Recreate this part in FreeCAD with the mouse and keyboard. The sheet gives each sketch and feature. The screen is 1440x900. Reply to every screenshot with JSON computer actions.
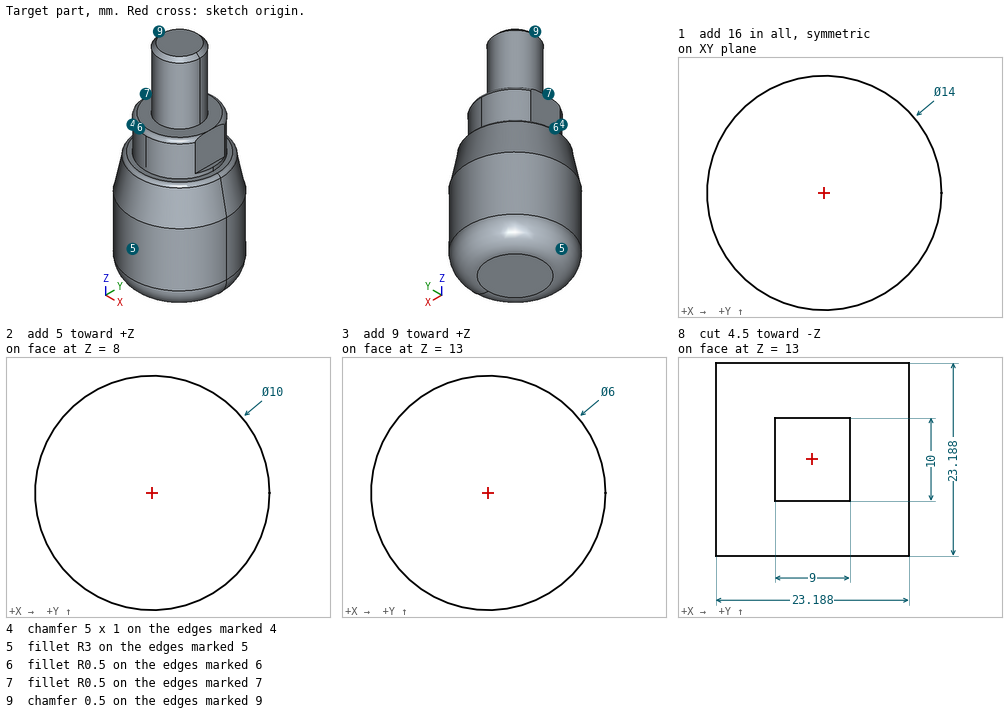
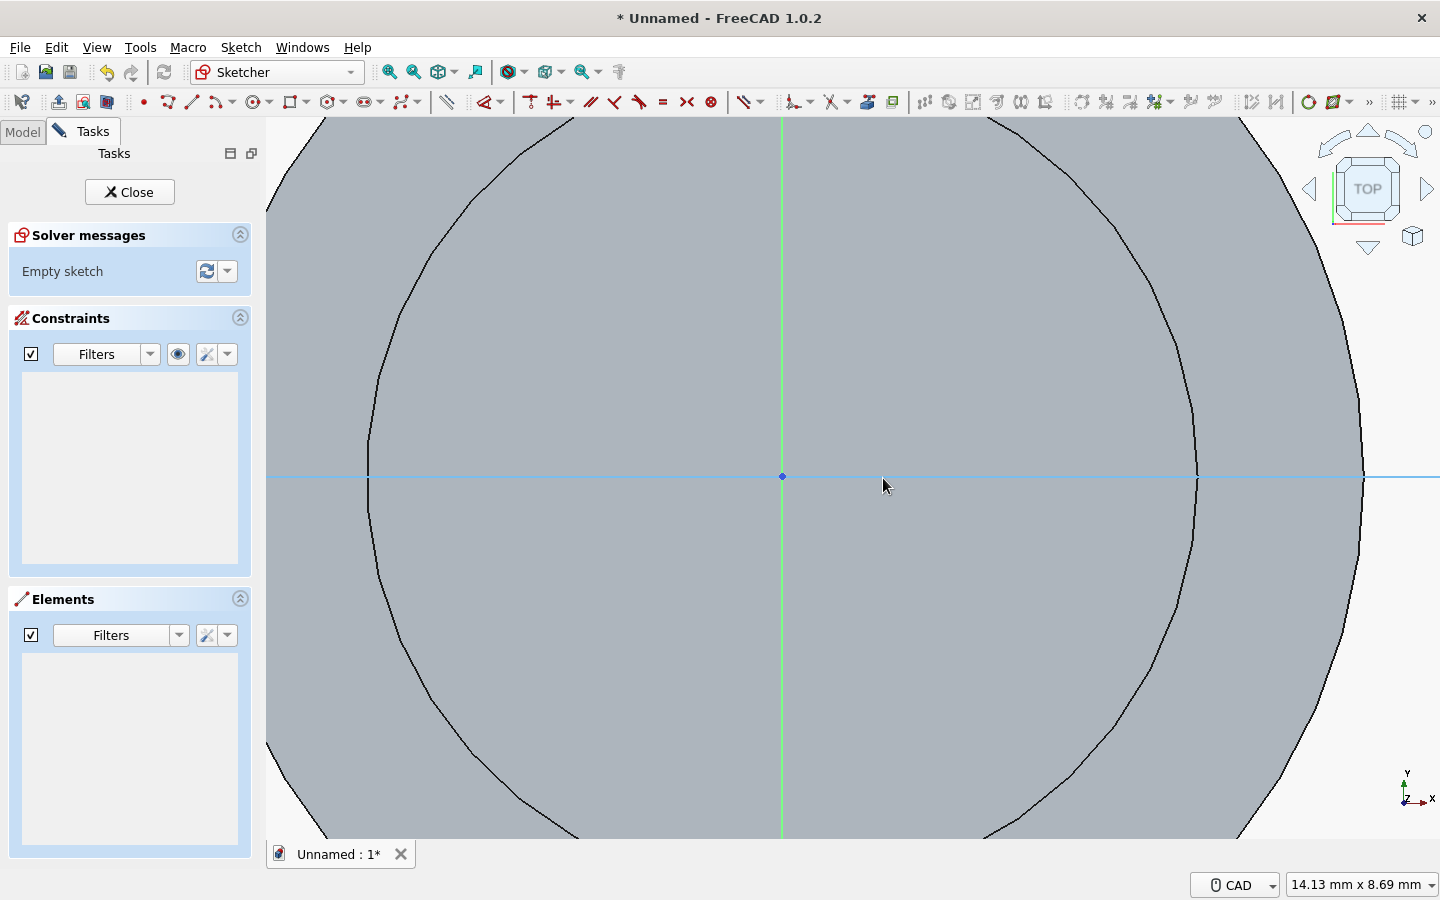
{"action": "key", "text": "g c"}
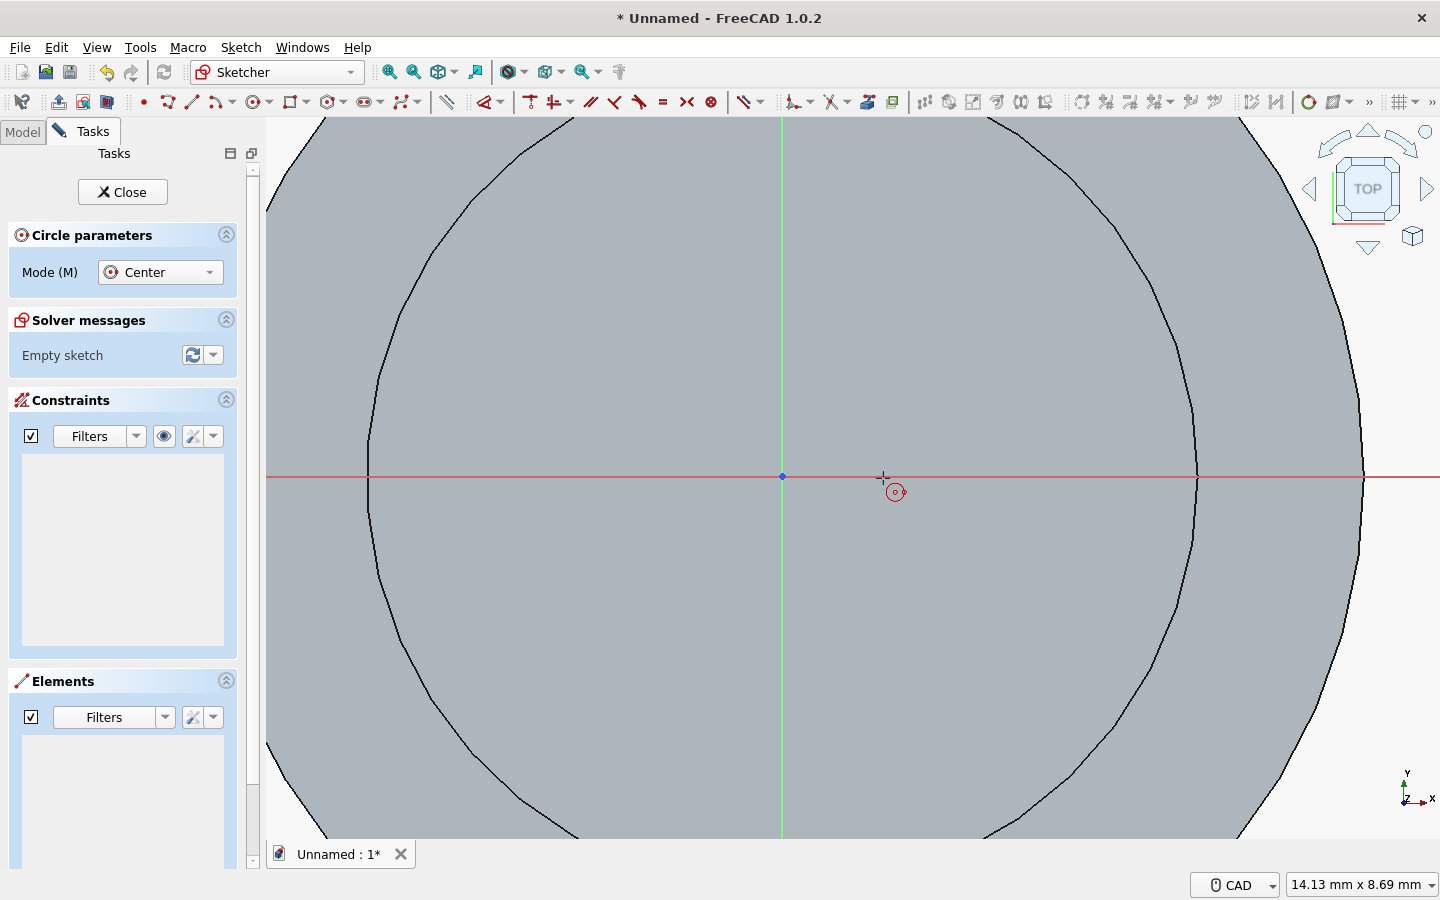
{"action": "left_click", "coordinate": [782, 477]}
{"action": "left_click", "coordinate": [958, 301]}
{"action": "key", "text": "Escape"}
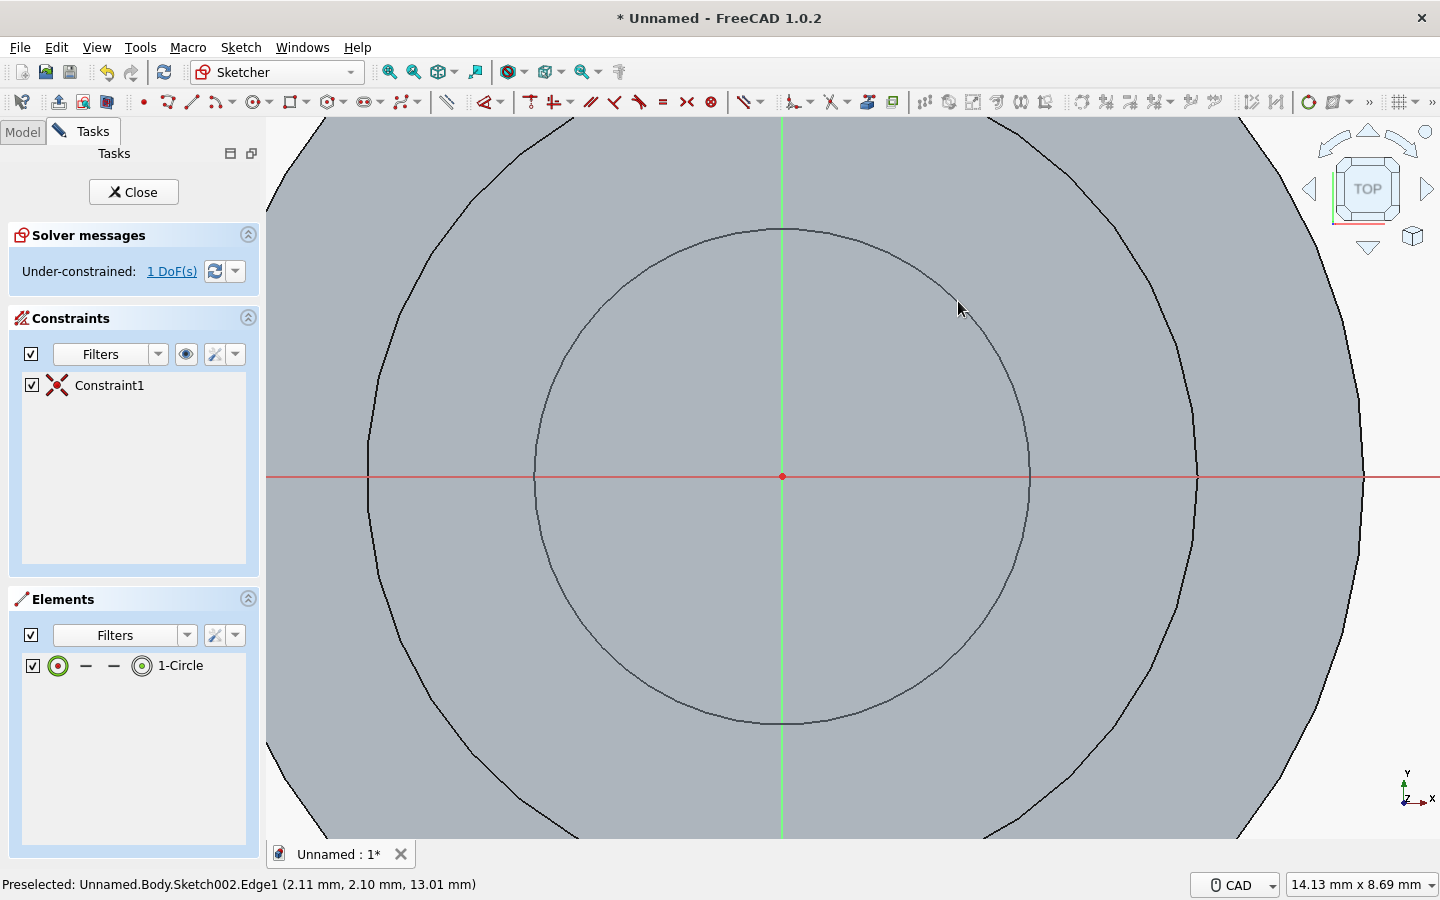
{"action": "left_click", "coordinate": [957, 301]}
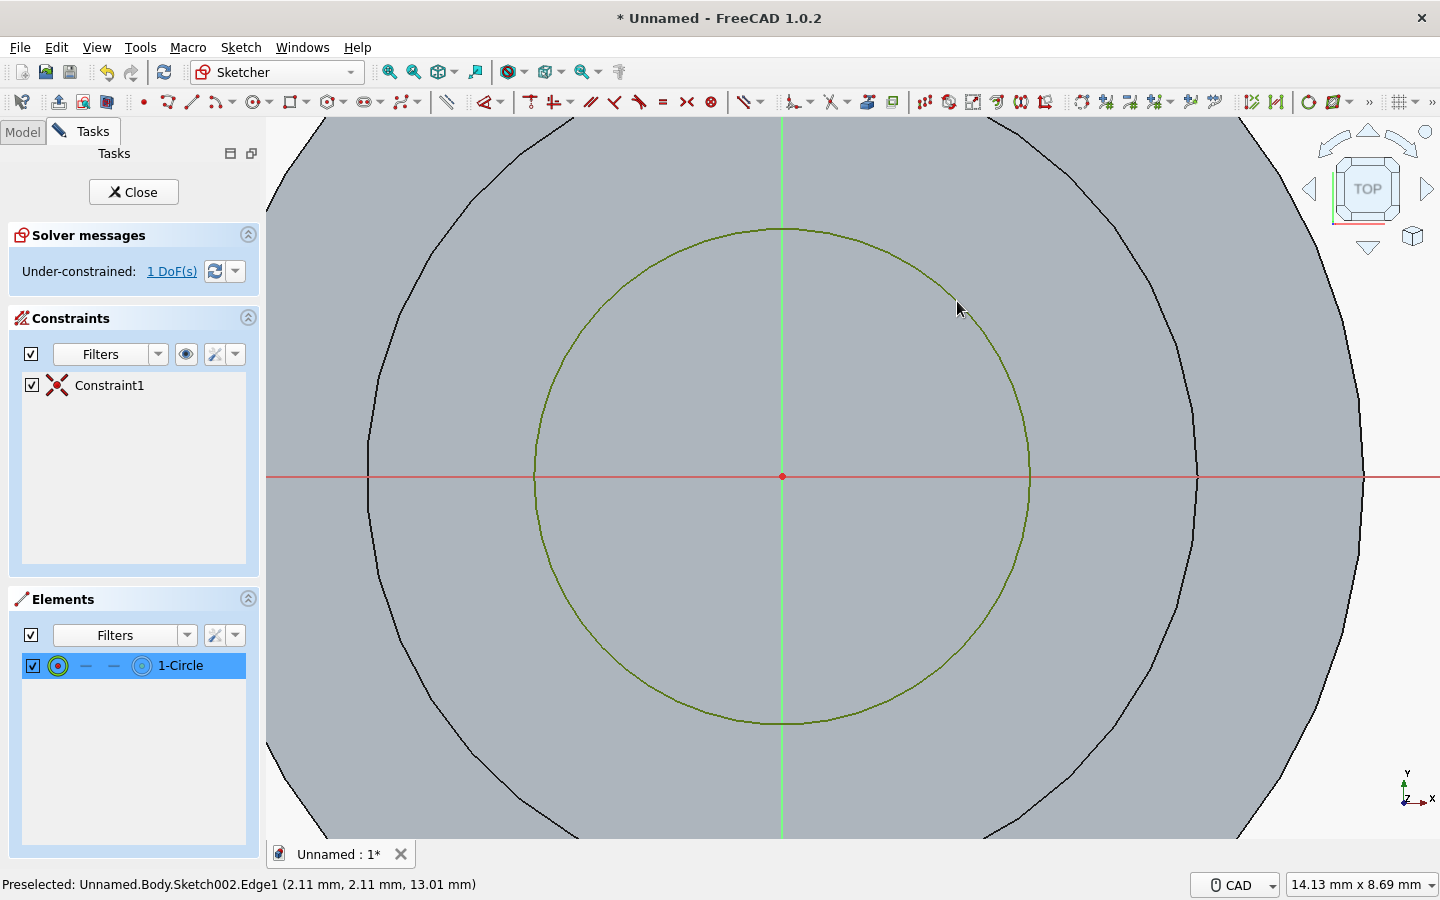
{"action": "key", "text": "k o"}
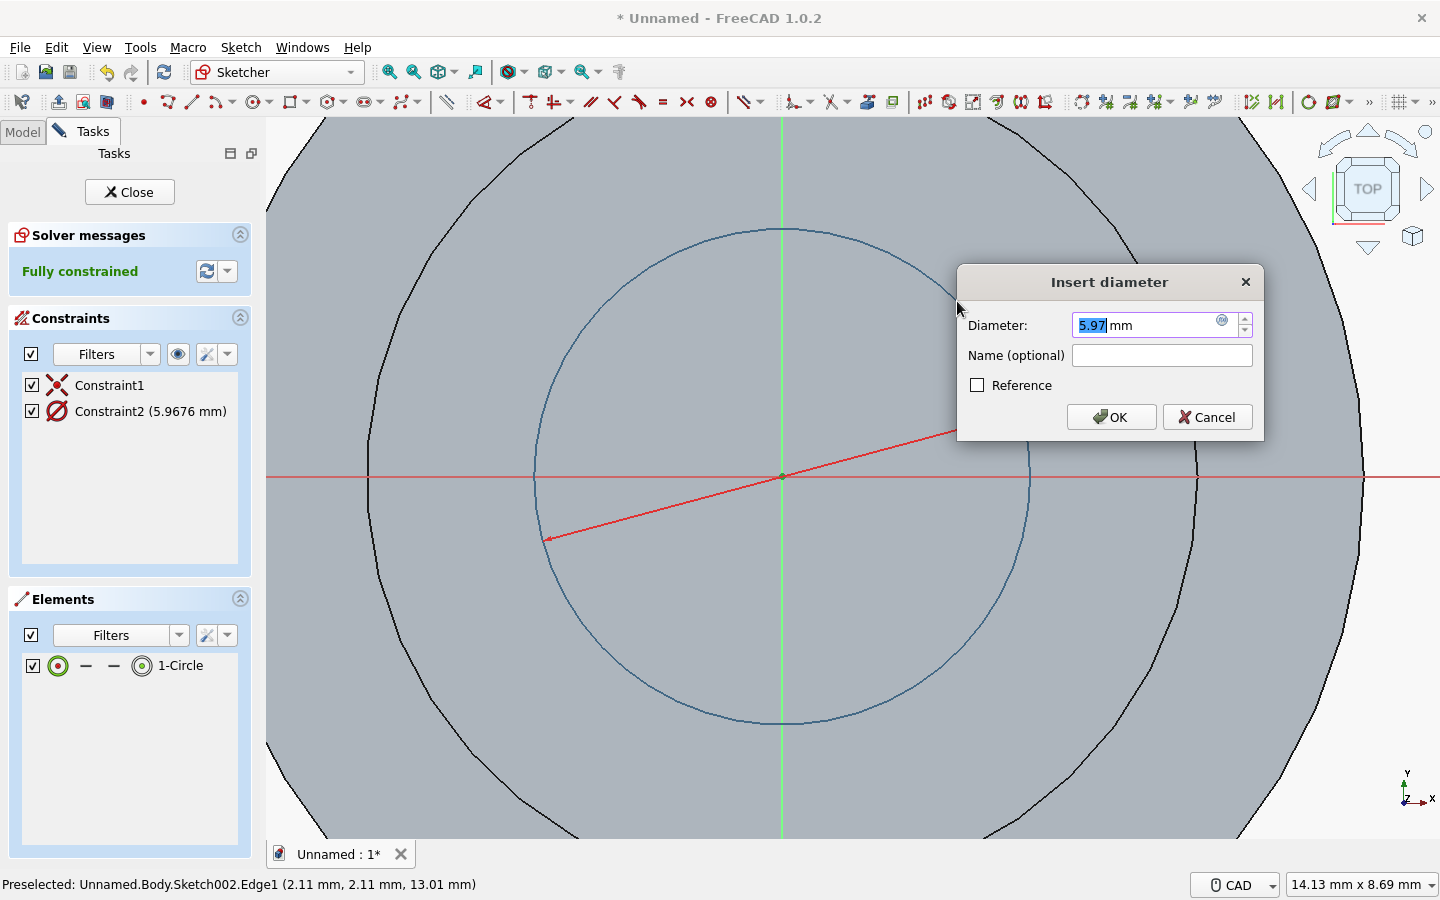
{"action": "type", "text": "6"}
{"action": "key", "text": "Return"}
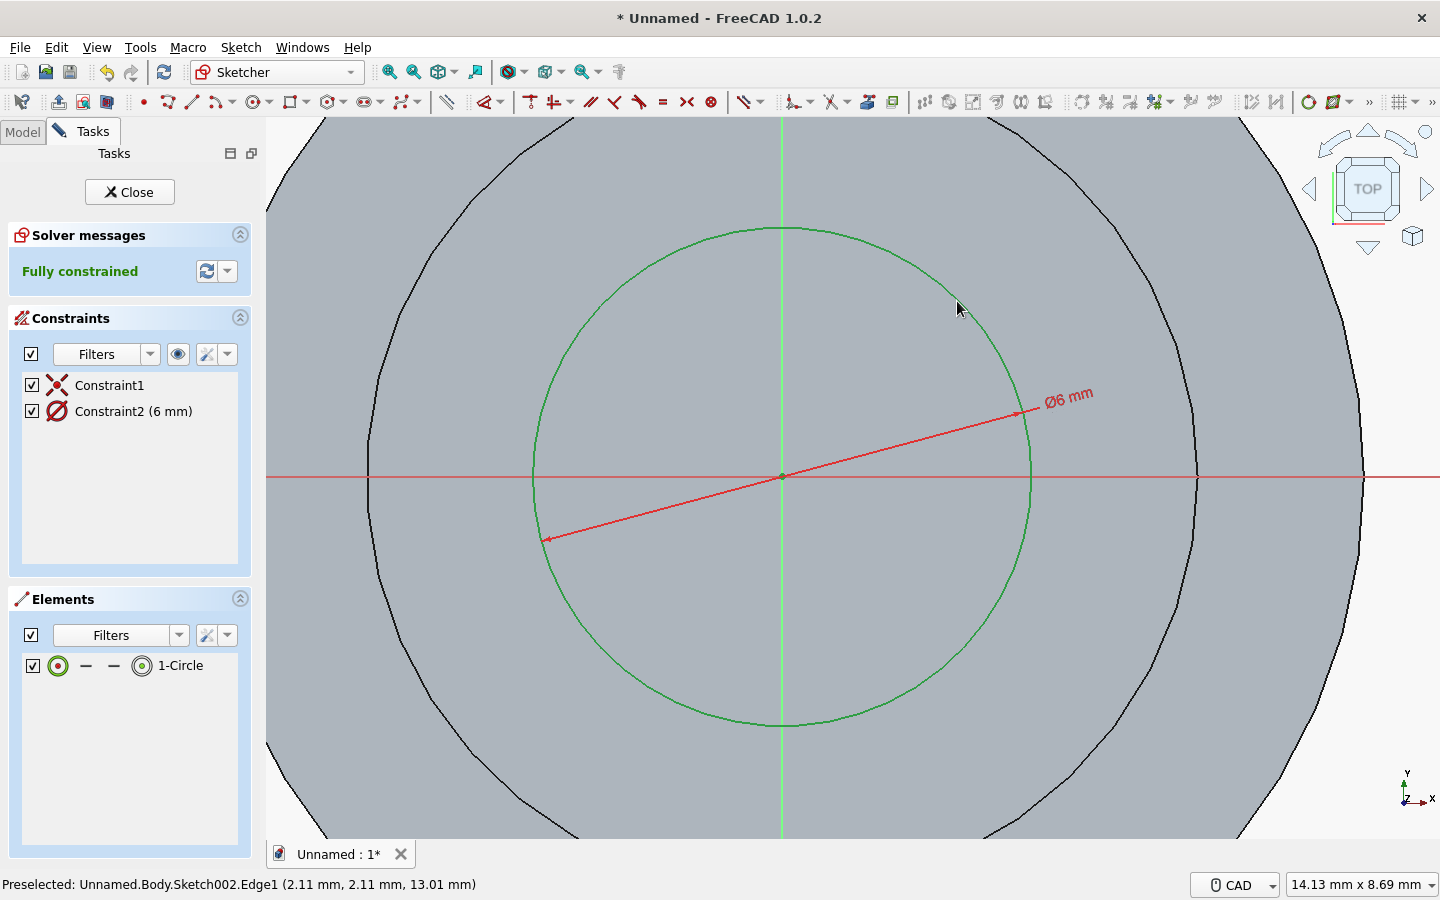
{"action": "left_click", "coordinate": [130, 192]}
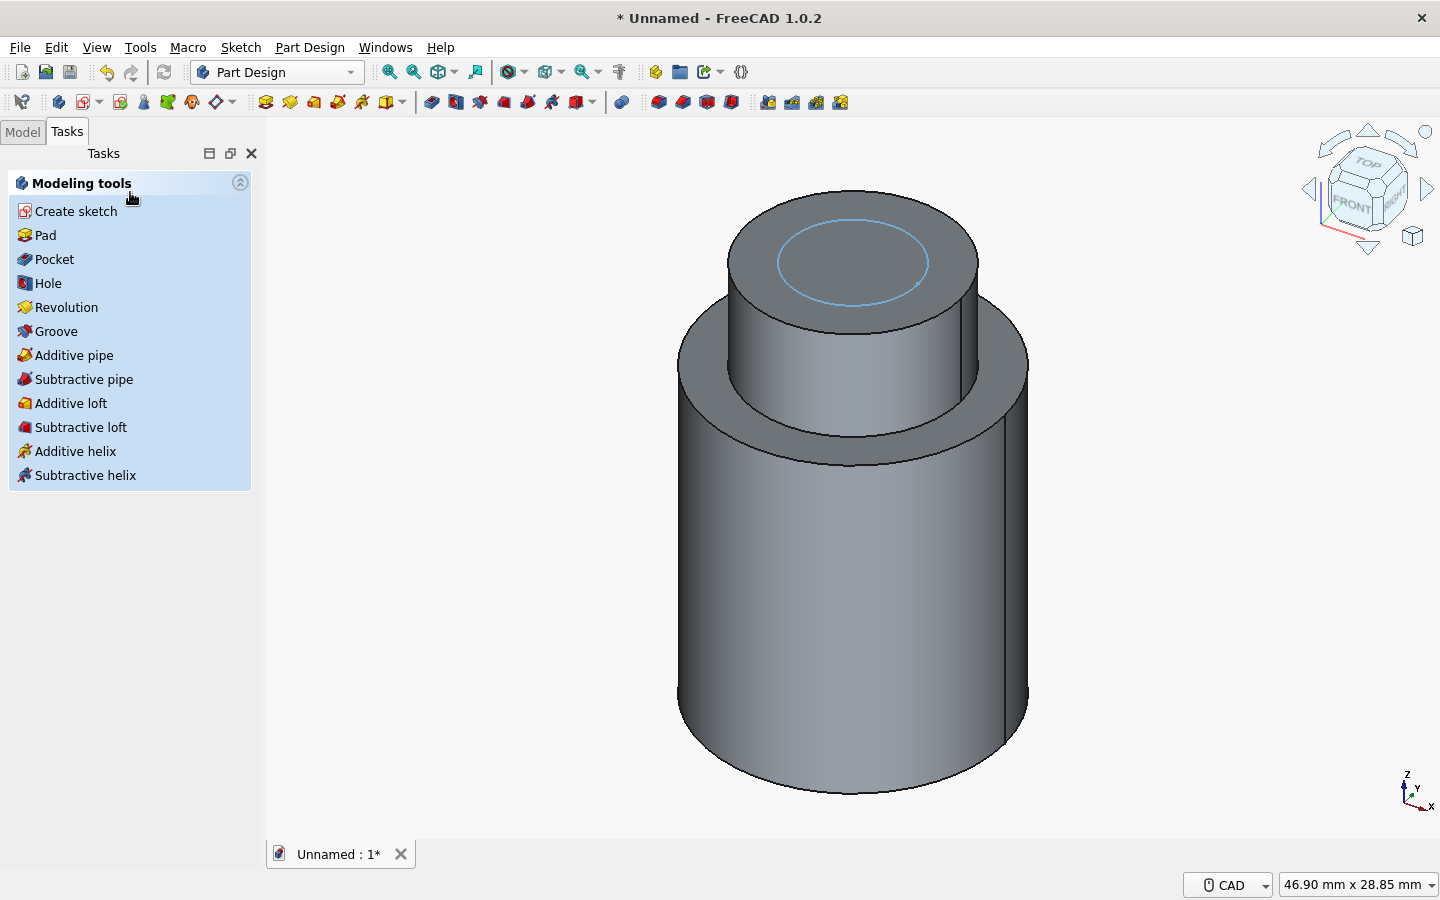
{"action": "left_click", "coordinate": [266, 102]}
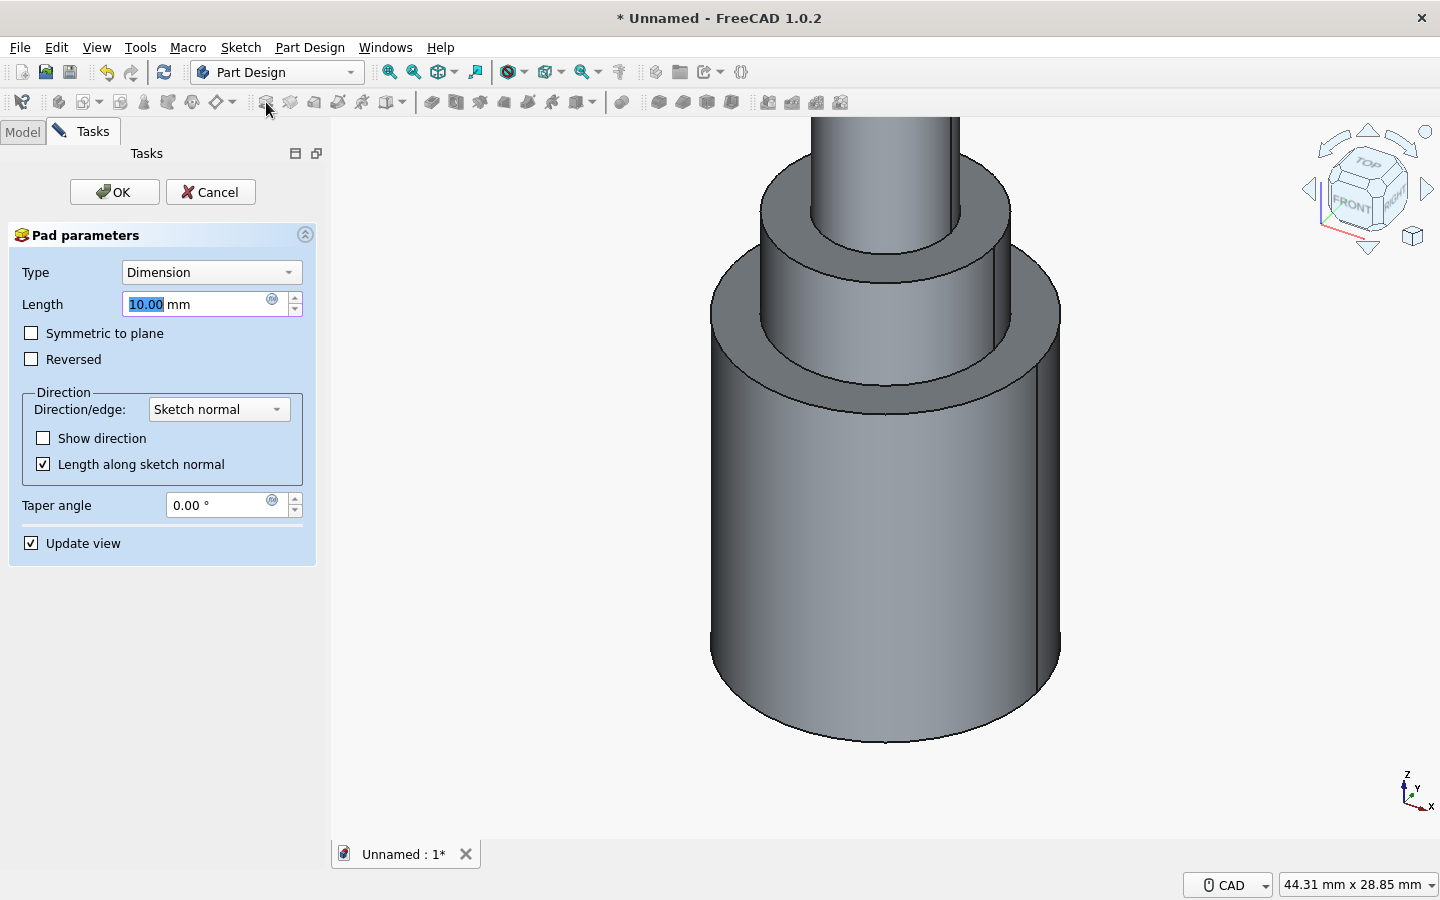
{"action": "type", "text": "9"}
{"action": "key", "text": "Tab"}